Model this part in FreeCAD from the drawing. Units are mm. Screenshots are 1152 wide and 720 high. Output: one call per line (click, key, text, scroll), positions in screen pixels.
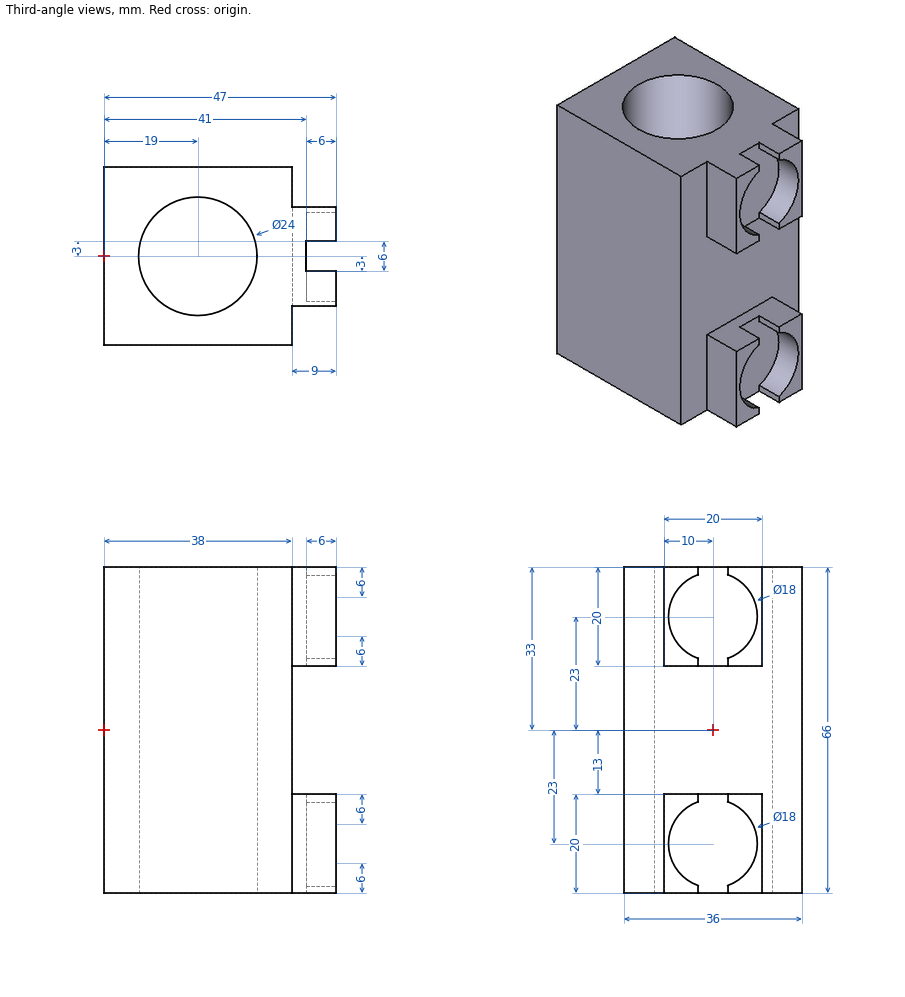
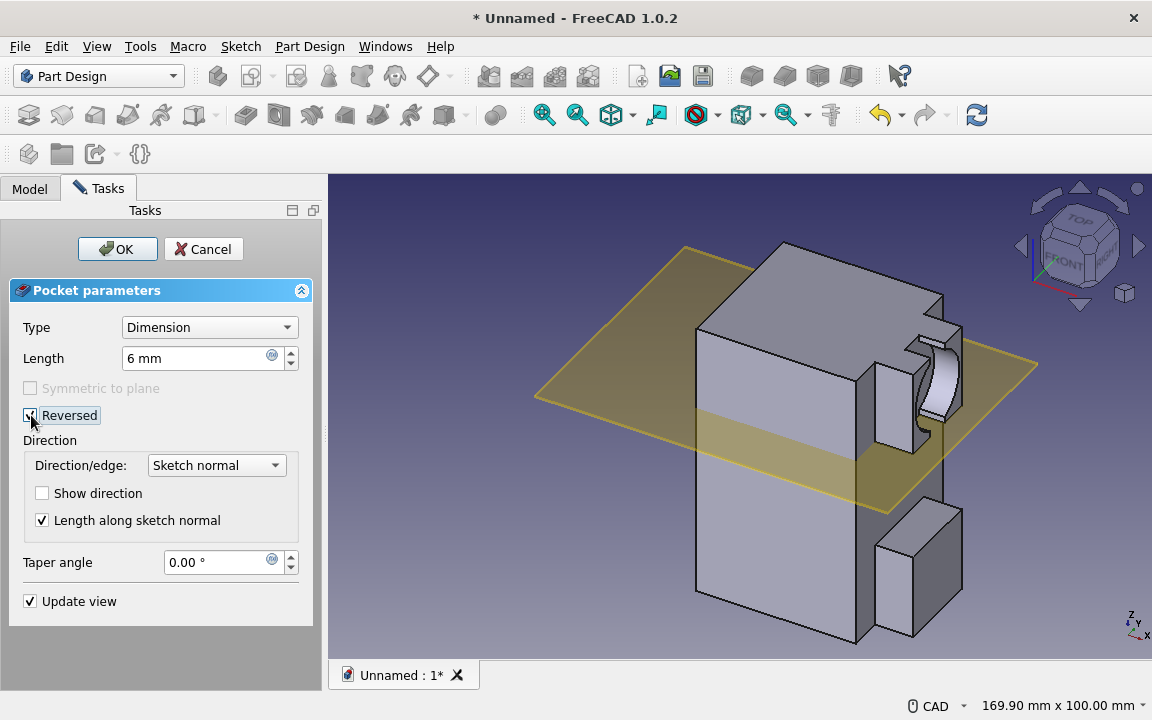
click(118, 249)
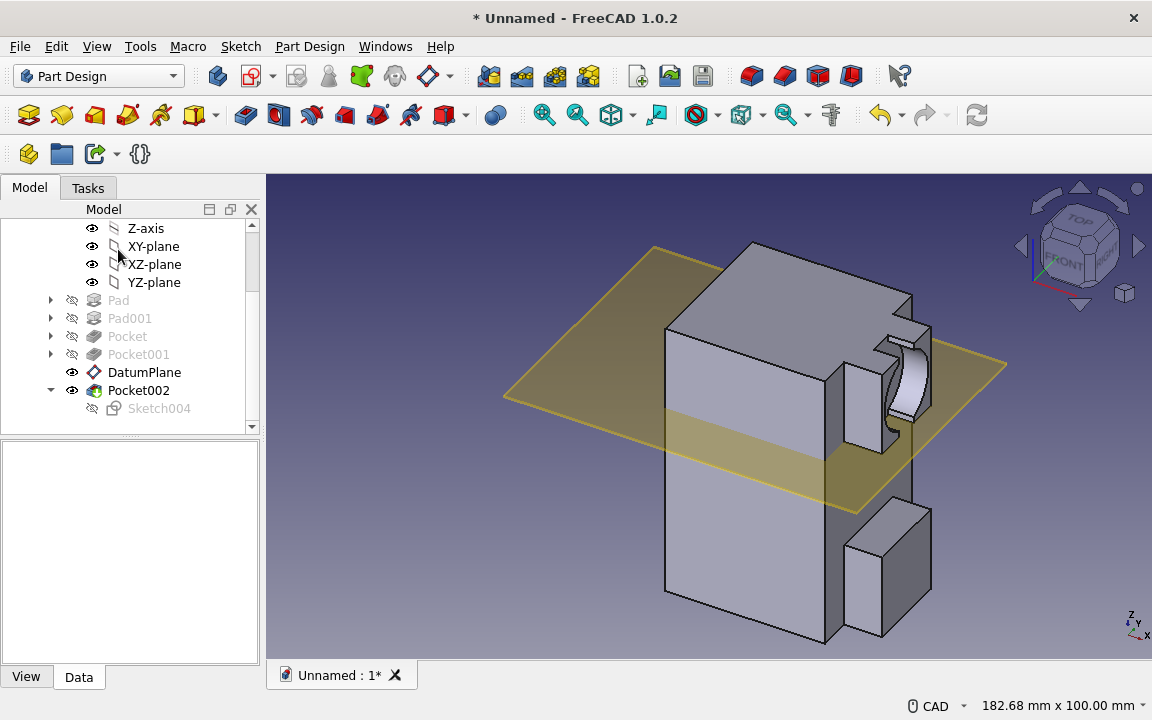
click(117, 372)
key(space)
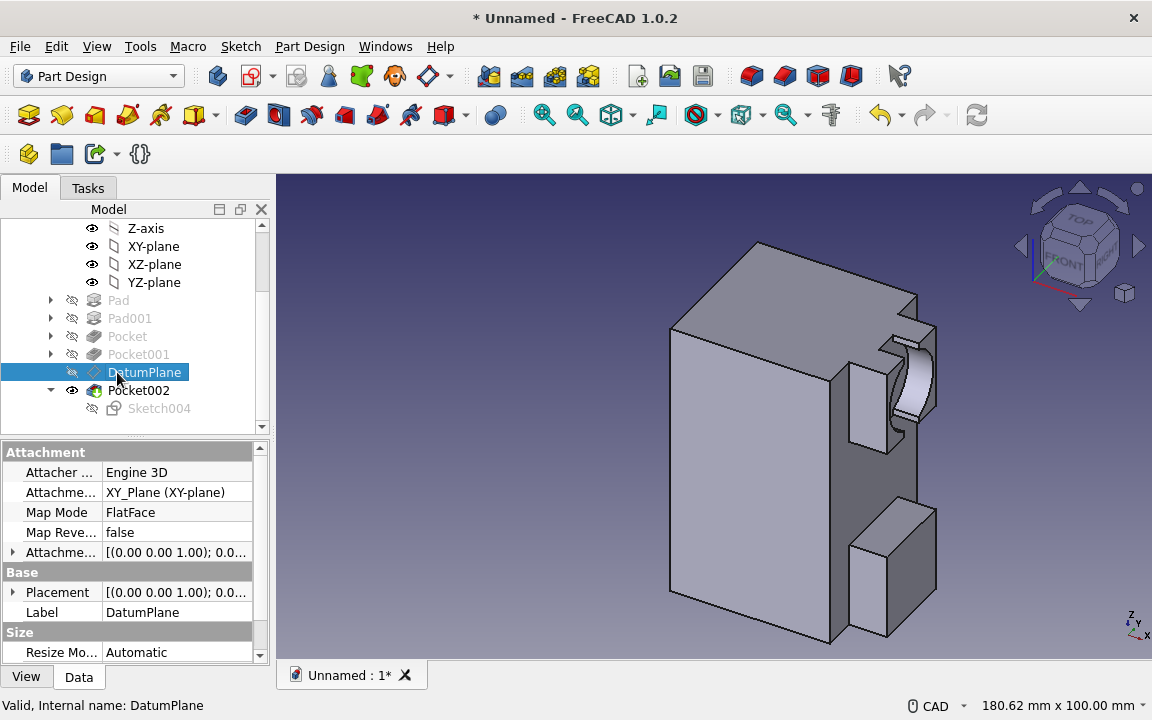
click(911, 572)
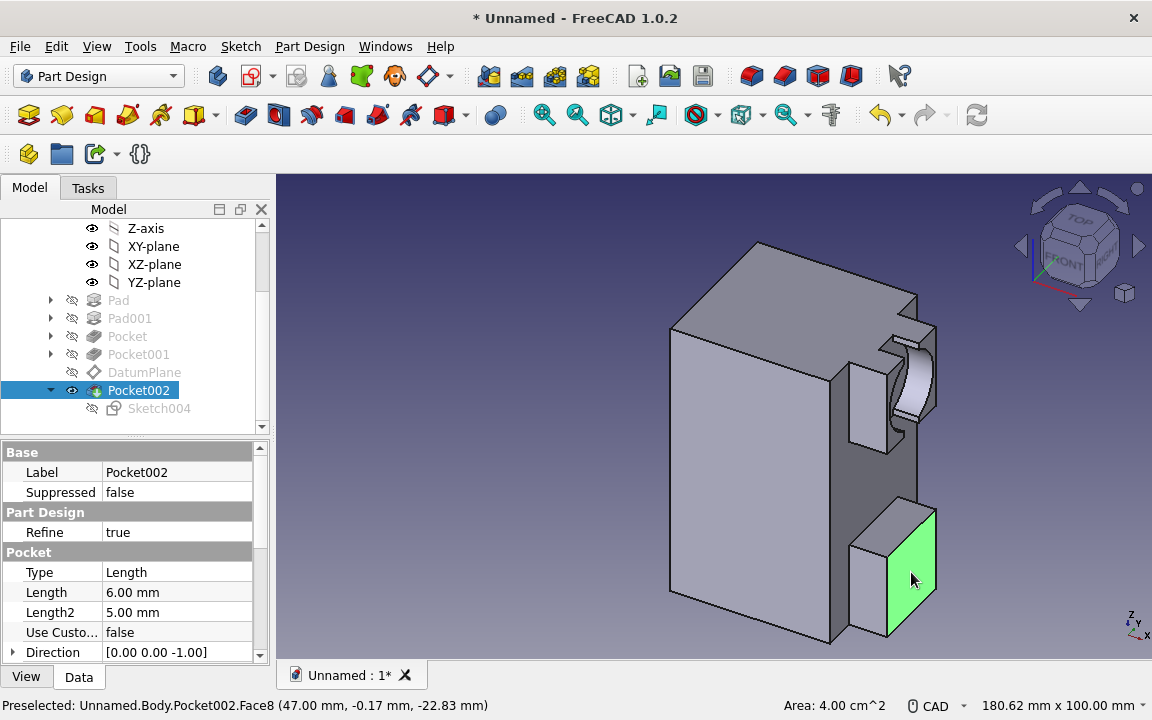
click(250, 76)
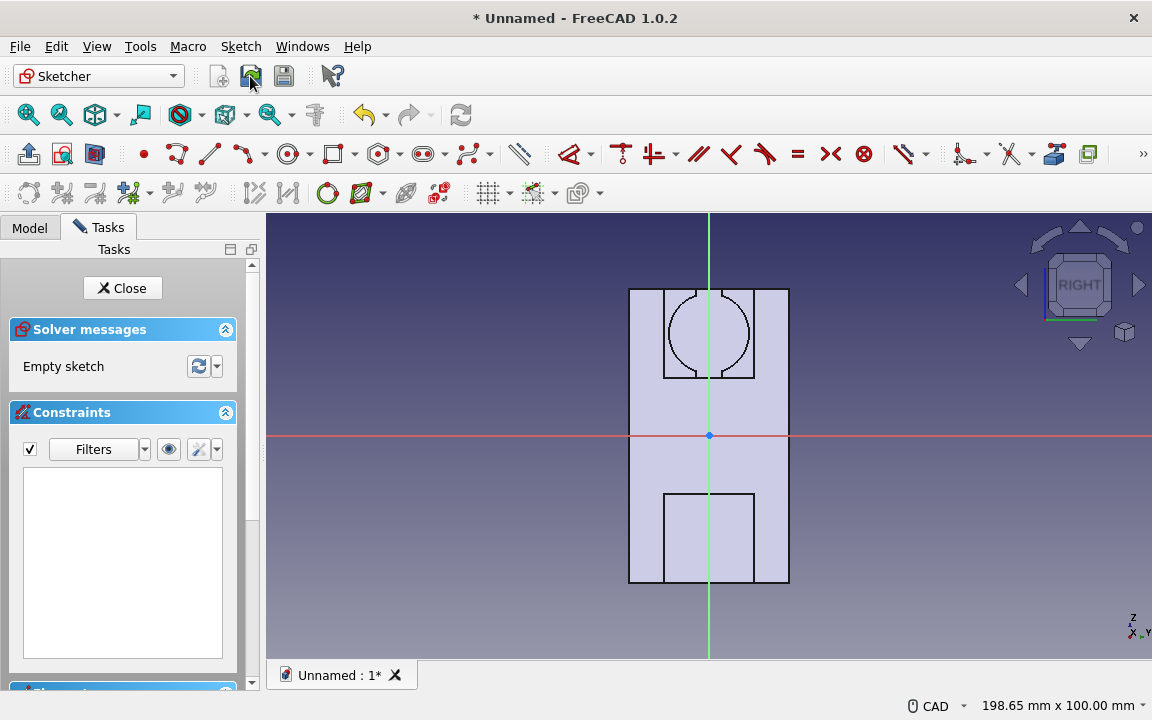
scroll(792, 594, up, 3)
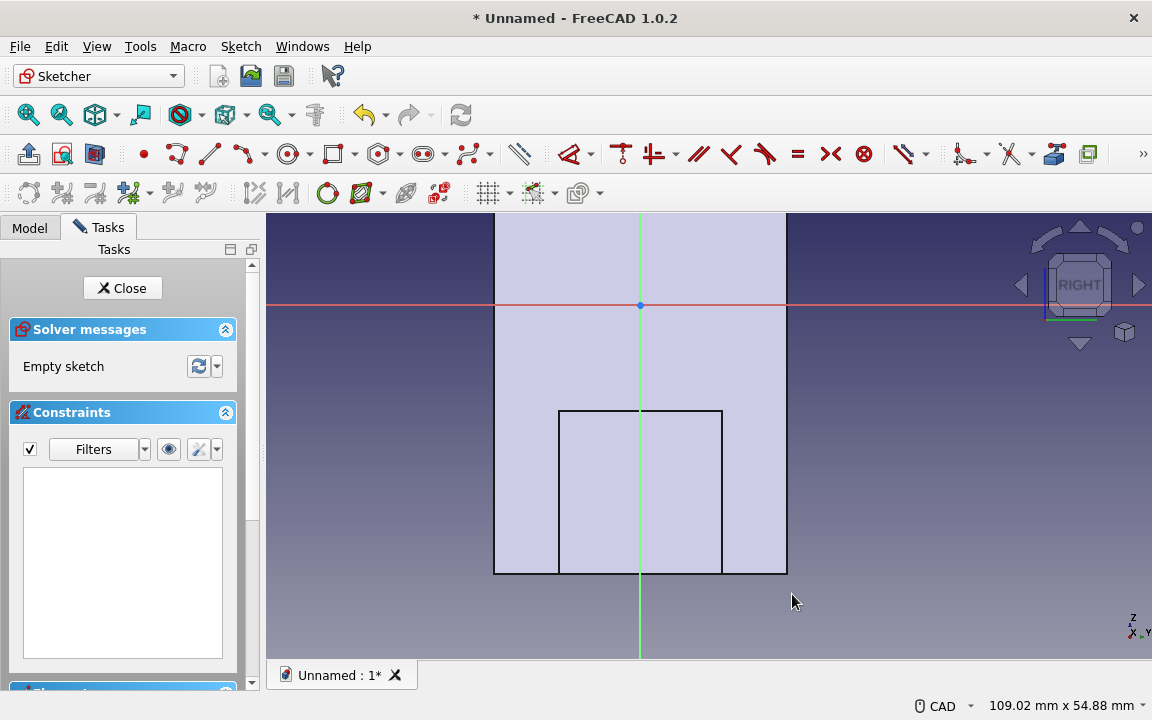
click(288, 154)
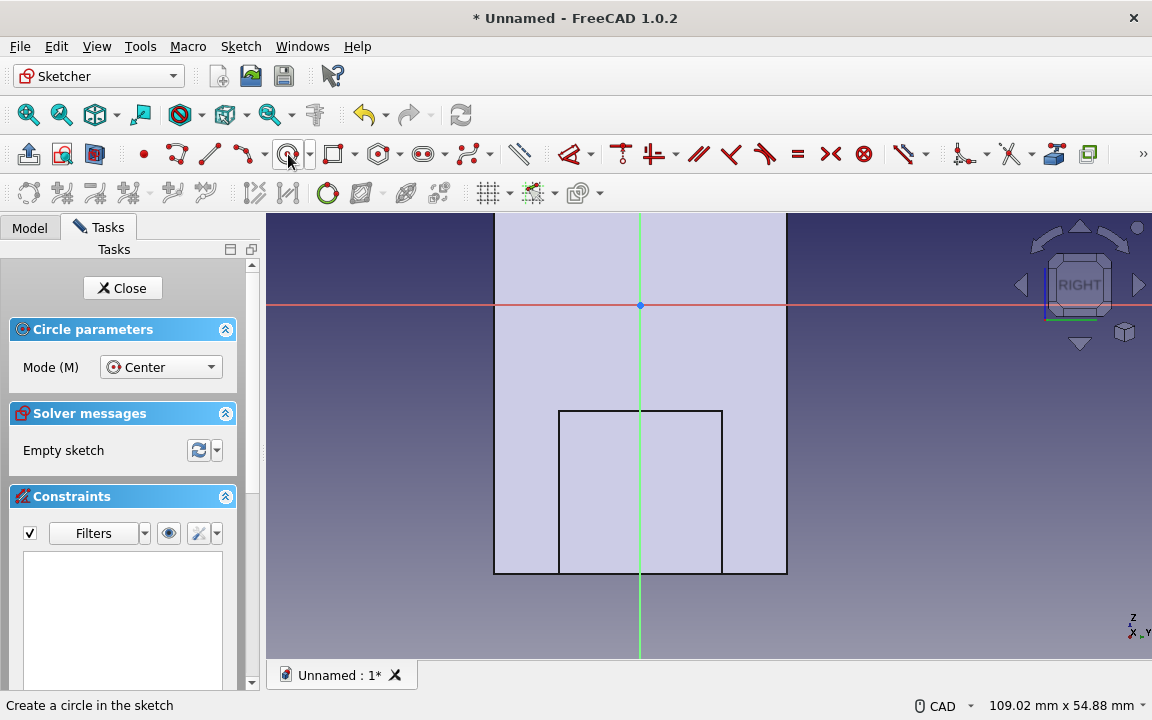
click(640, 492)
click(692, 441)
key(Escape)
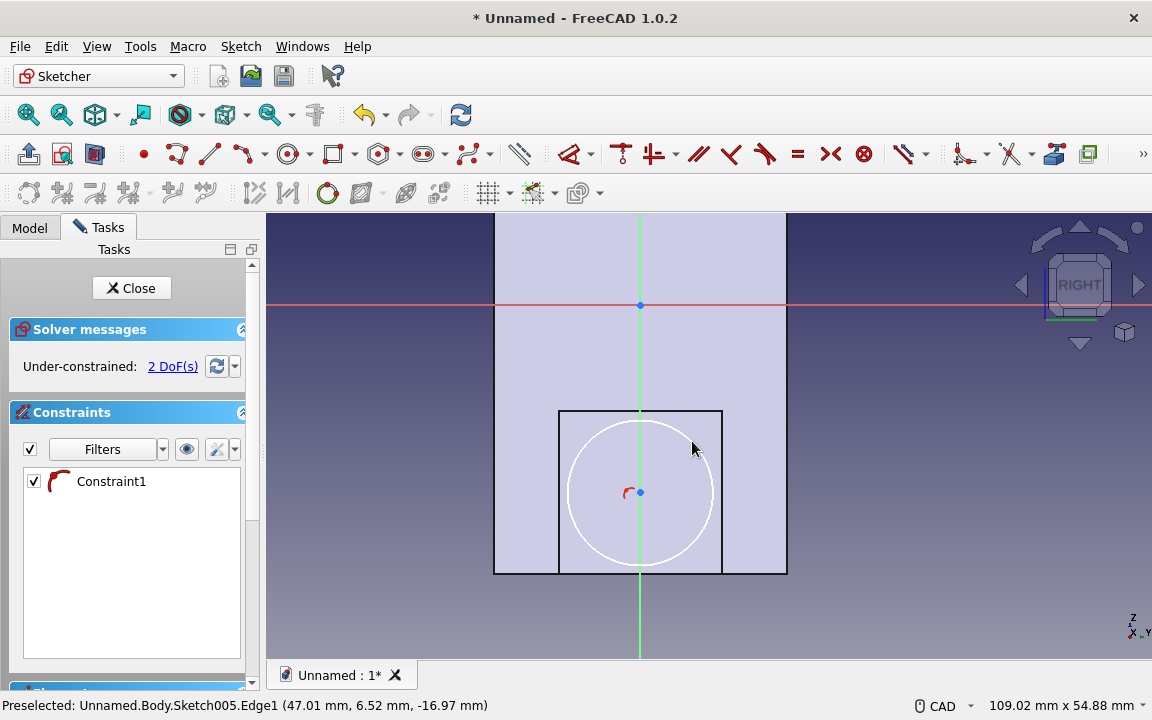
click(568, 154)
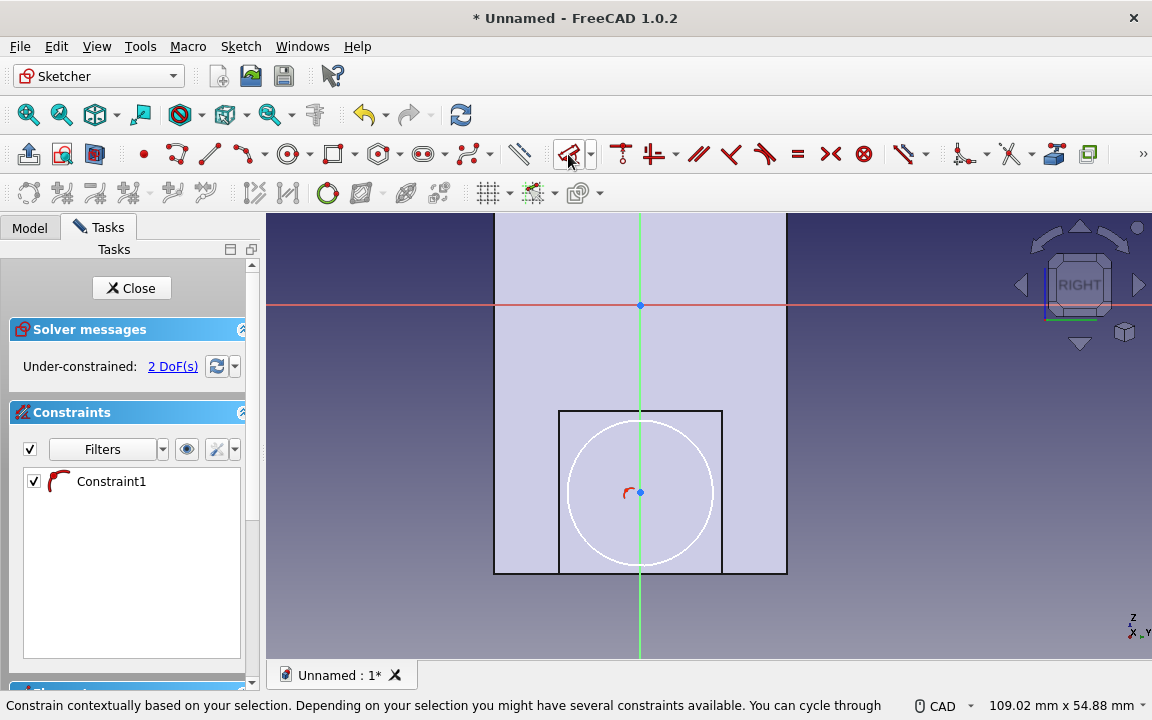
click(691, 441)
click(713, 418)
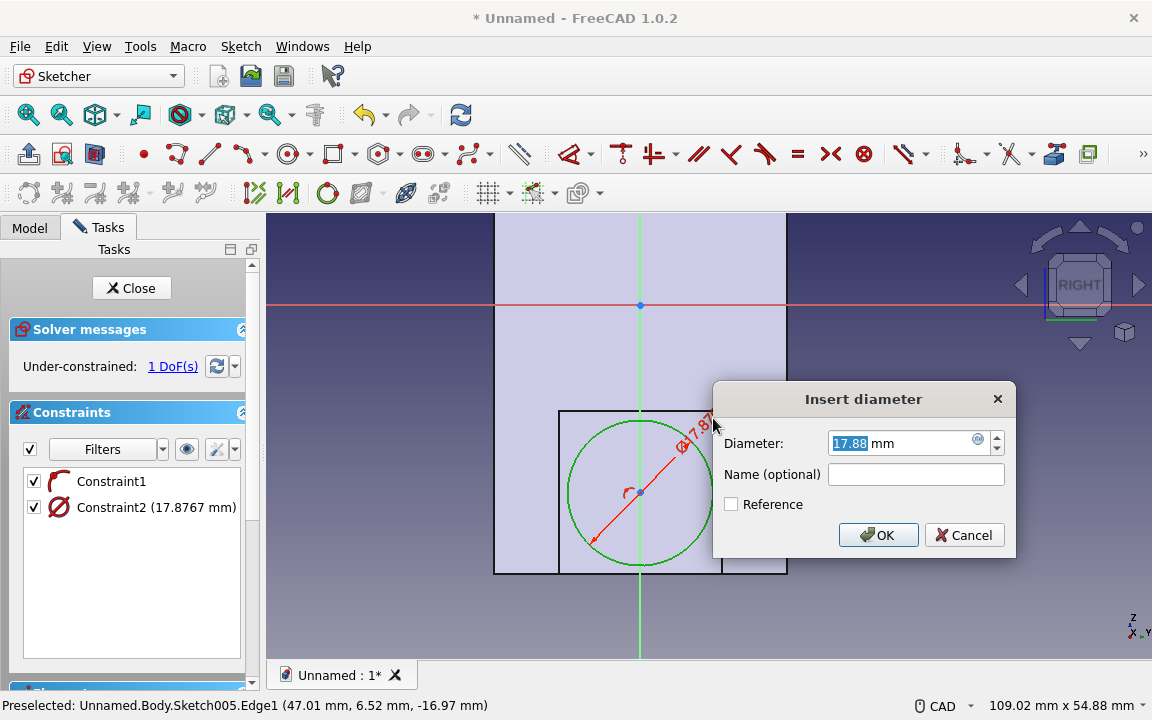
text(18)
key(Return)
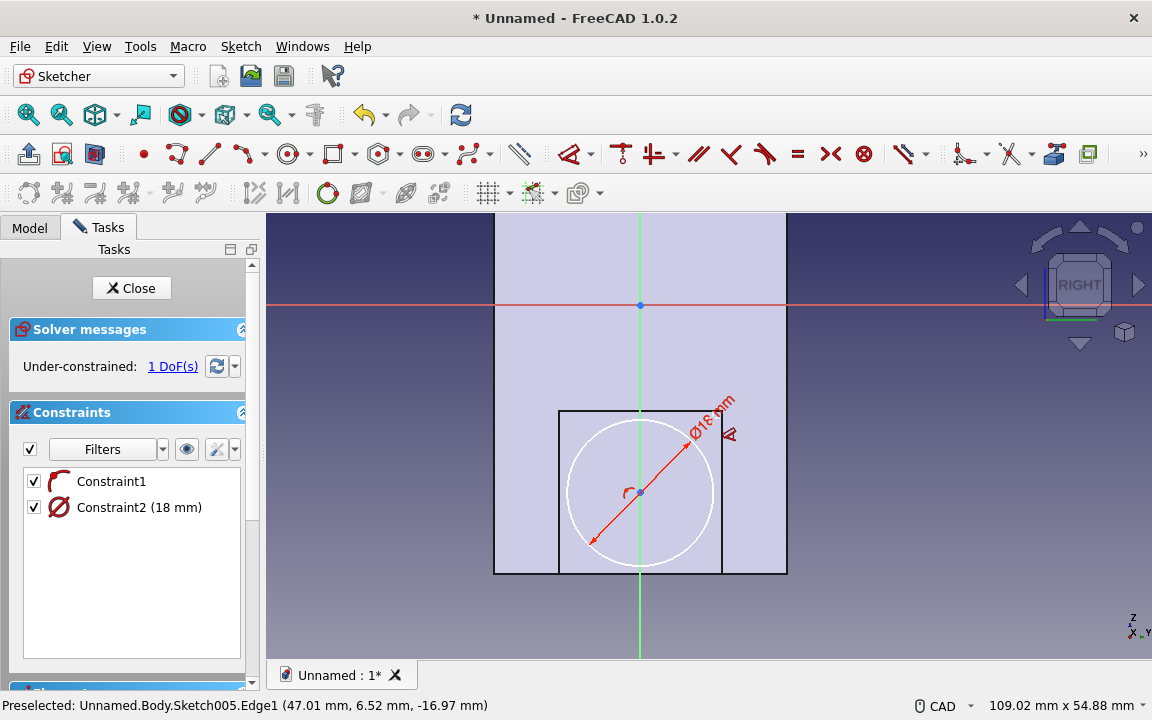
click(640, 493)
click(674, 356)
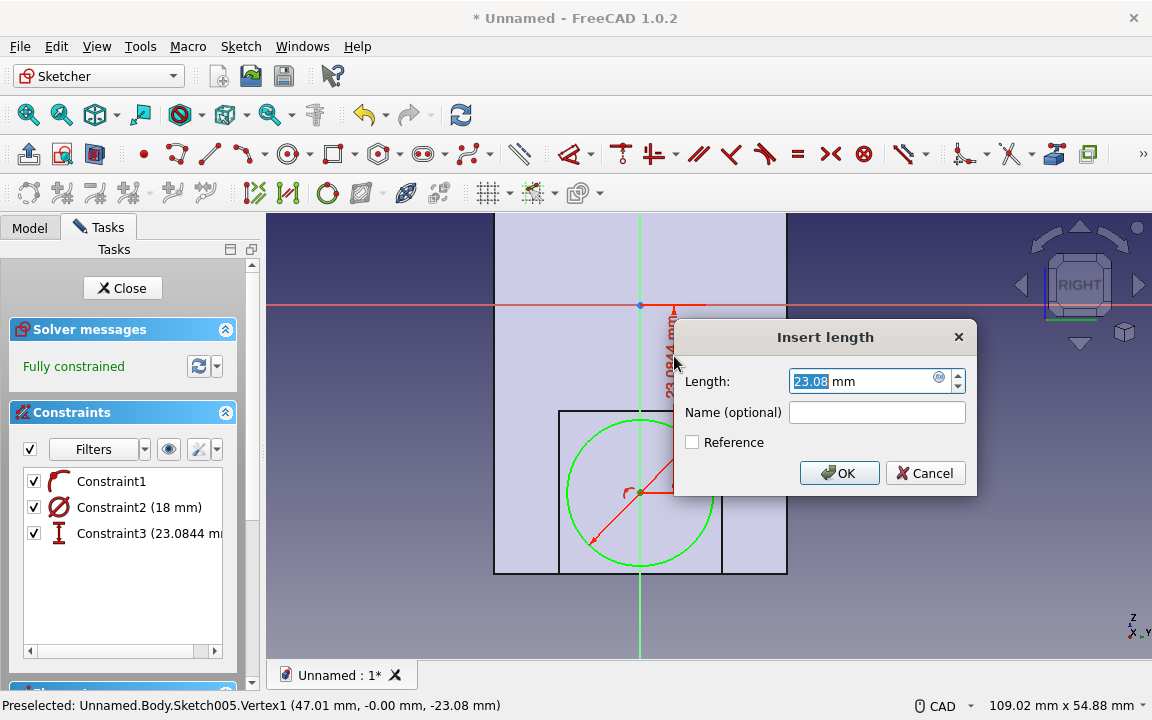
text(23)
key(Return)
key(Escape)